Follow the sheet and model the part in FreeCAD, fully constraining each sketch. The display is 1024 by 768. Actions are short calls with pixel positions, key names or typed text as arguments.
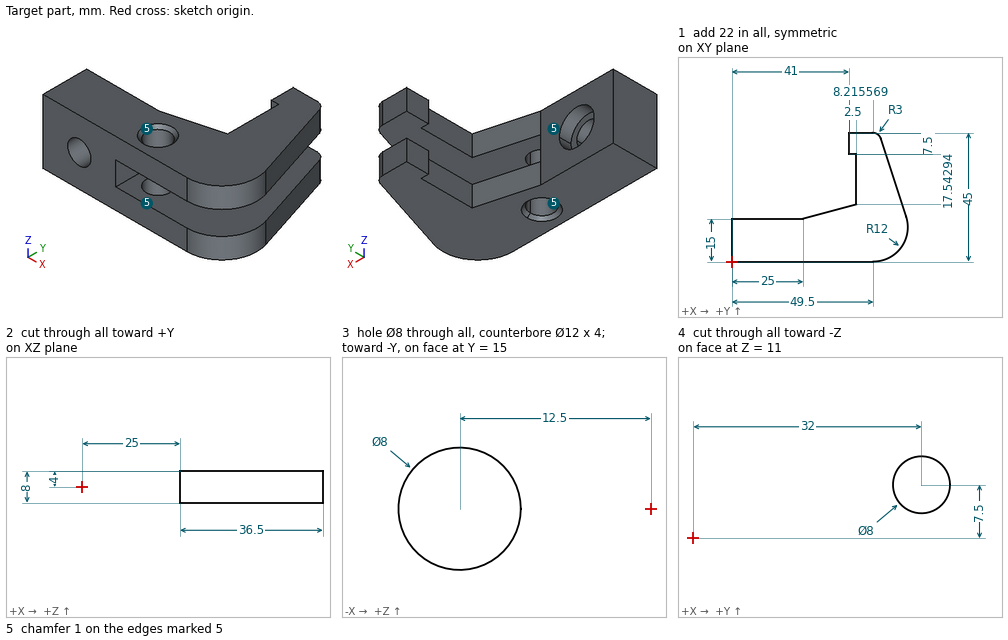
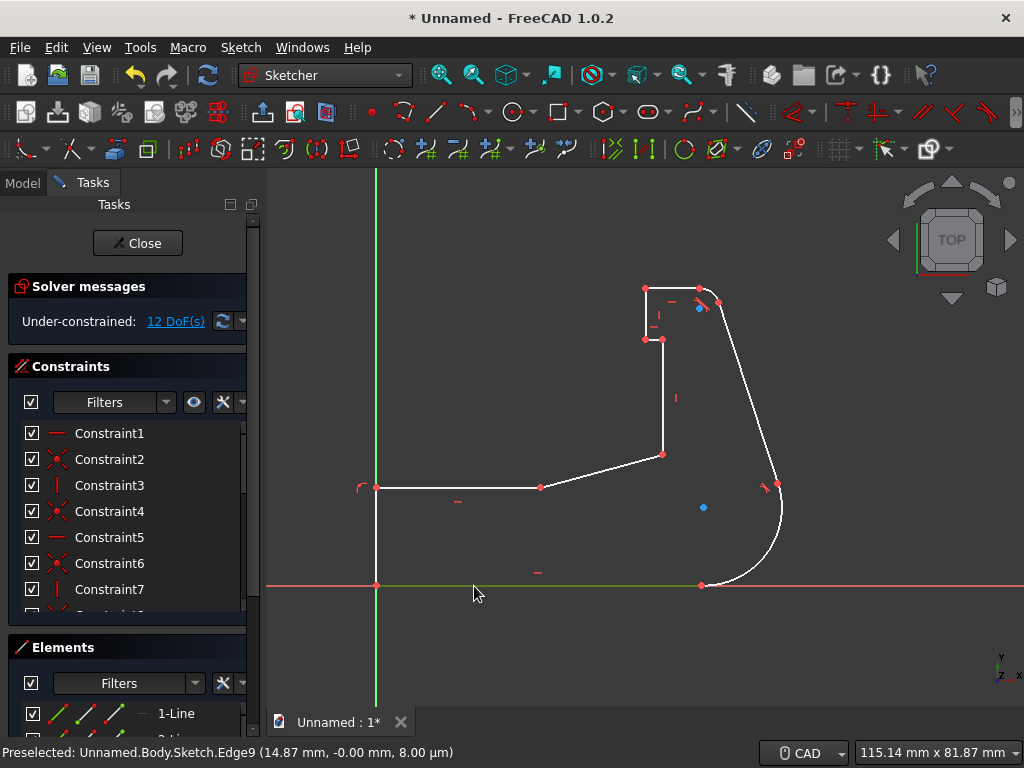
click(745, 574)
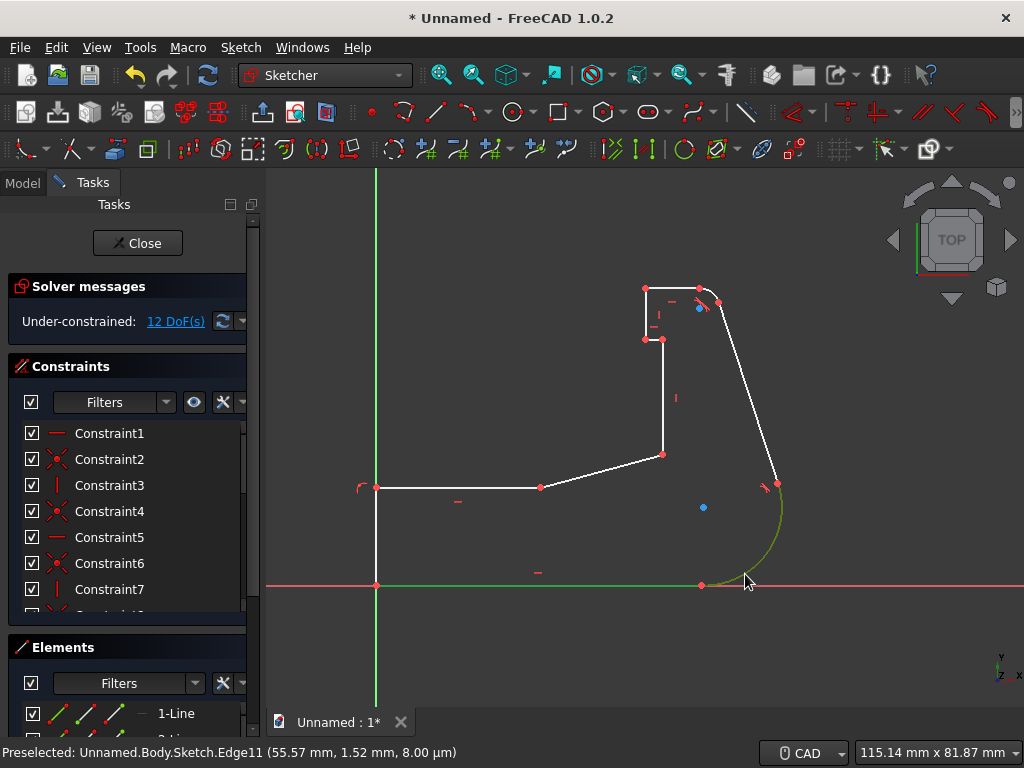
key(t)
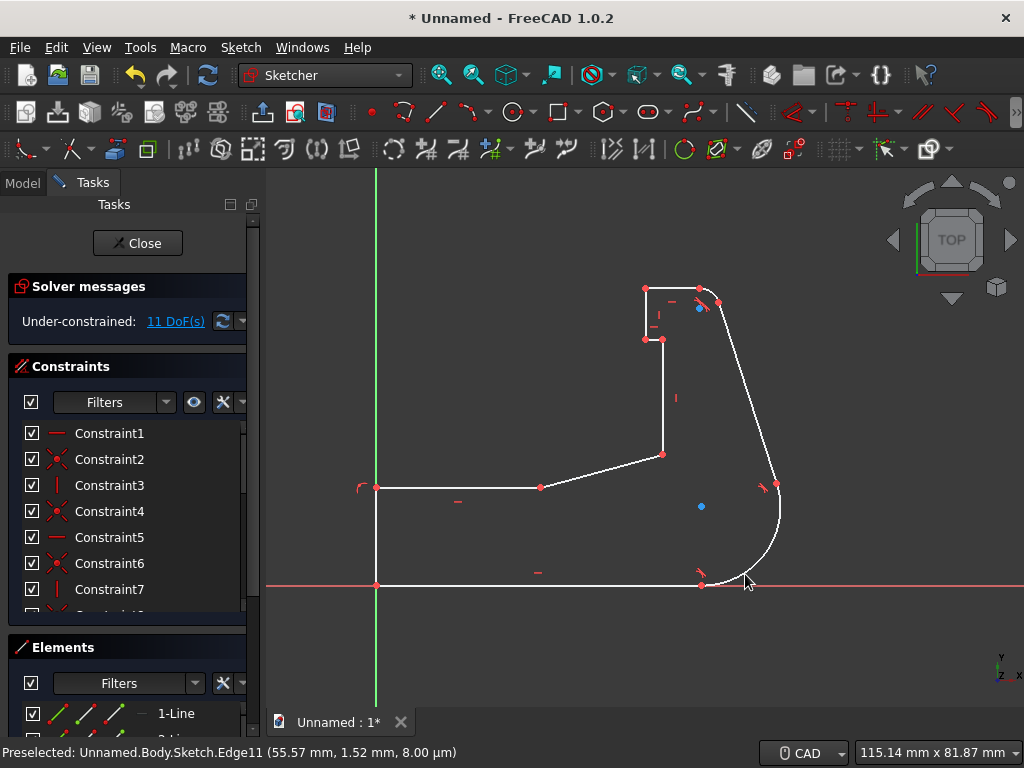
click(792, 112)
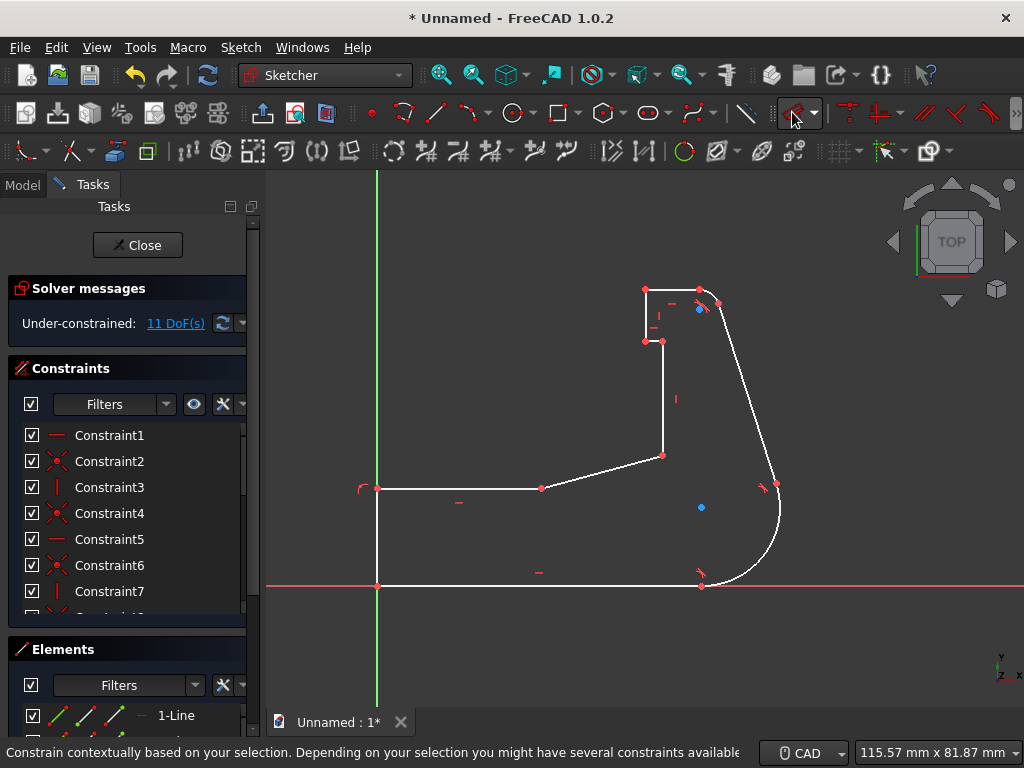
scroll(711, 294, up, 4)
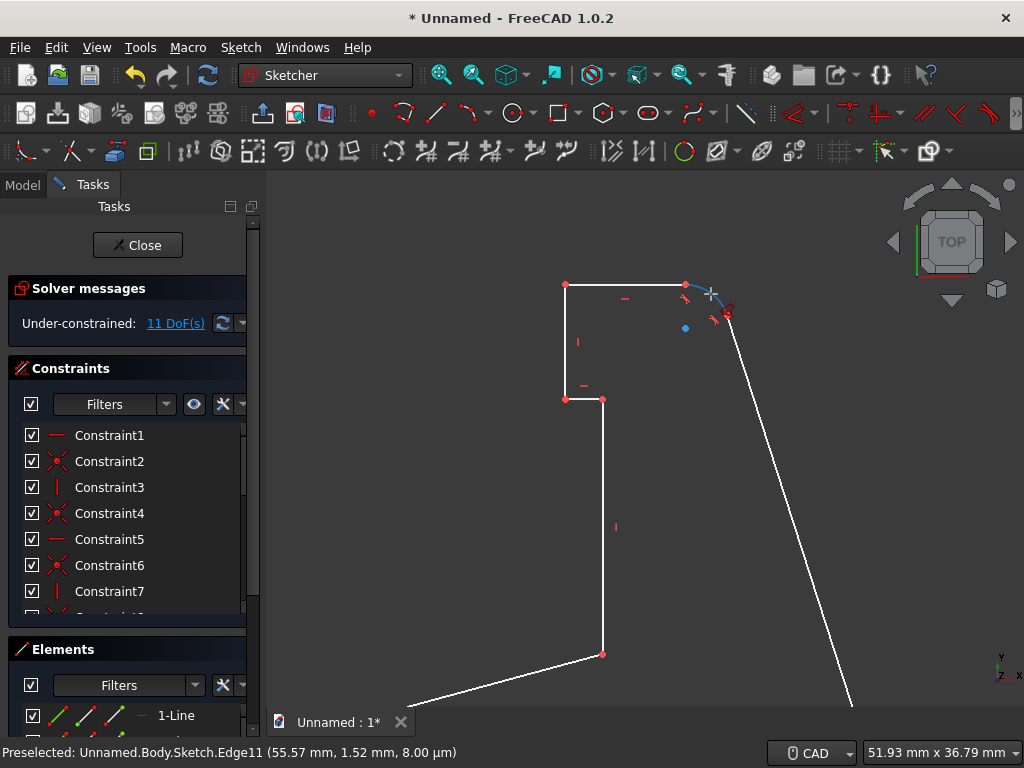
click(711, 293)
click(730, 267)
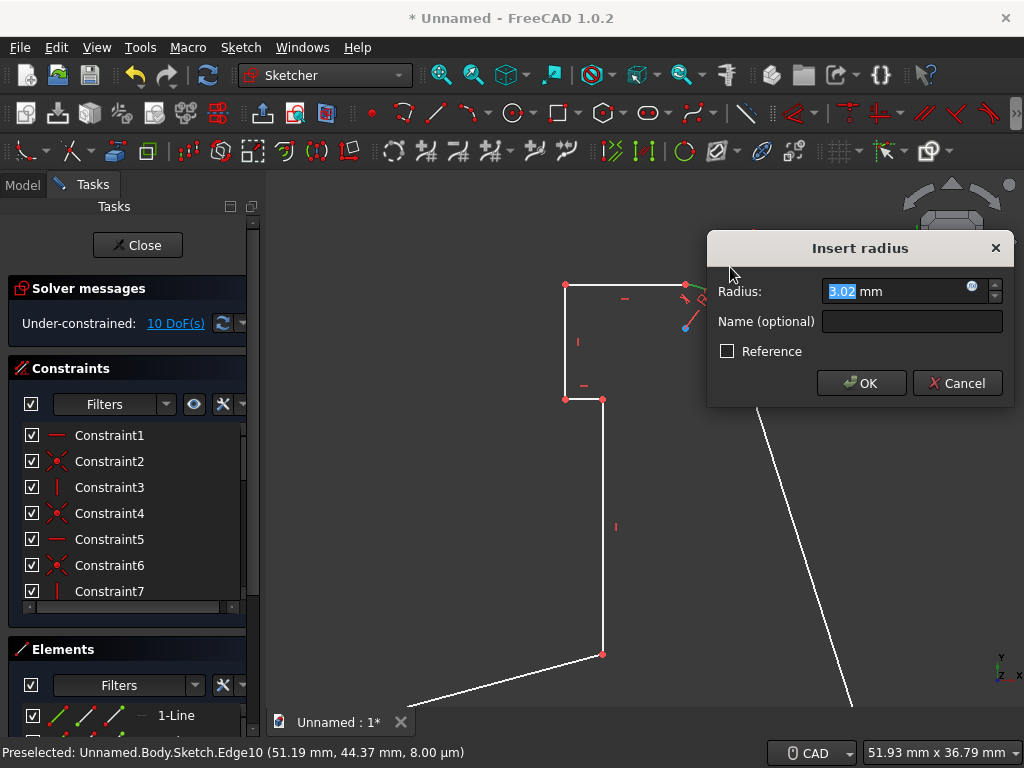
text(3)
key(Return)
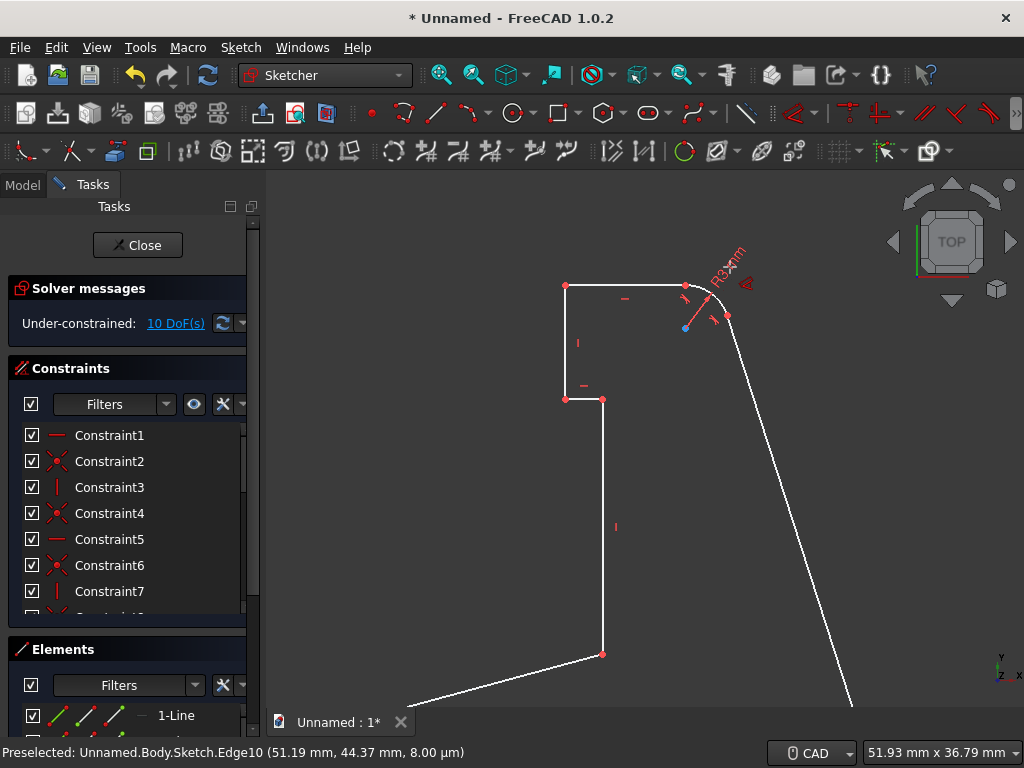
scroll(711, 294, down, 4)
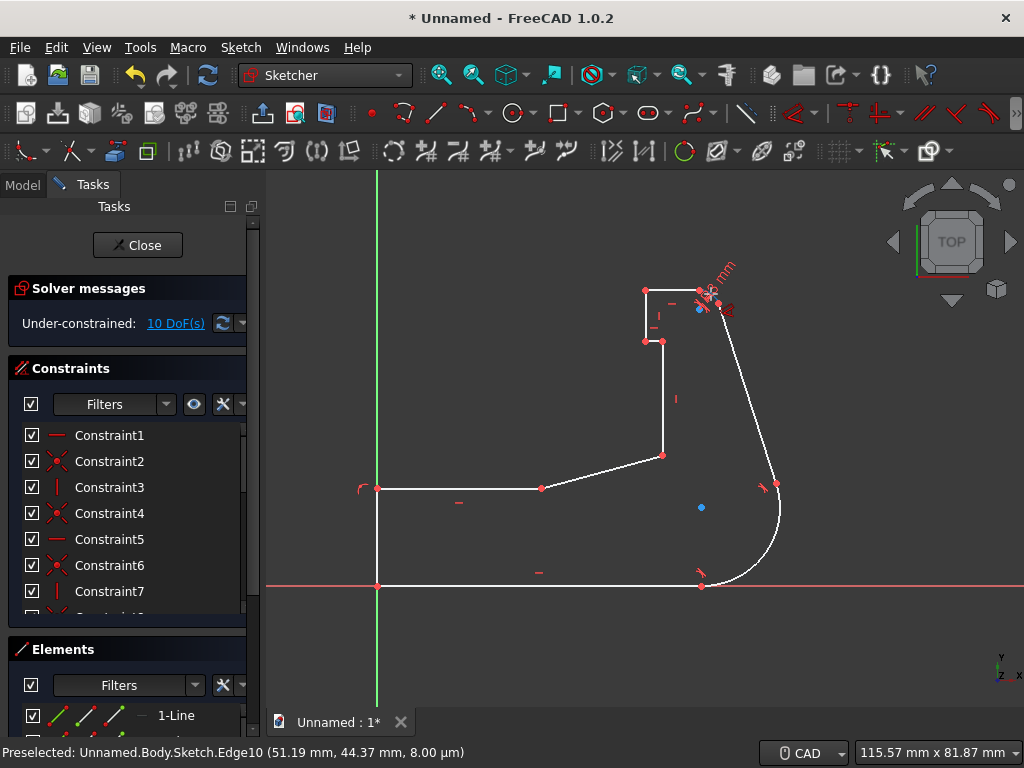
click(743, 574)
click(760, 601)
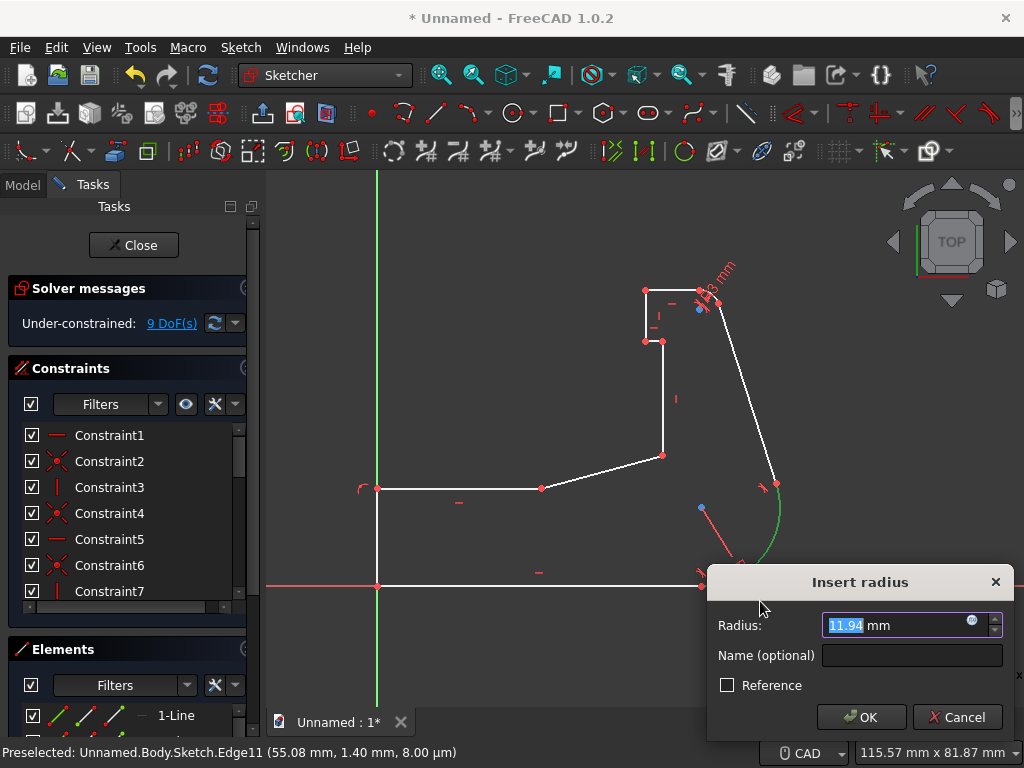
text(12)
key(Return)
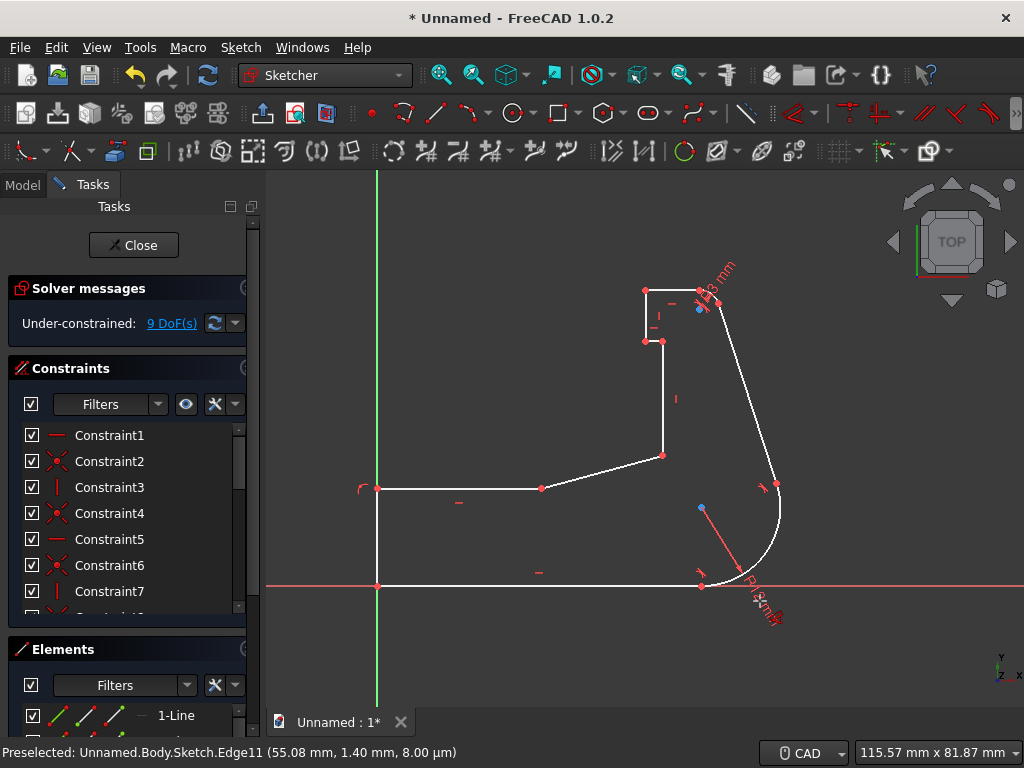
click(492, 489)
click(459, 523)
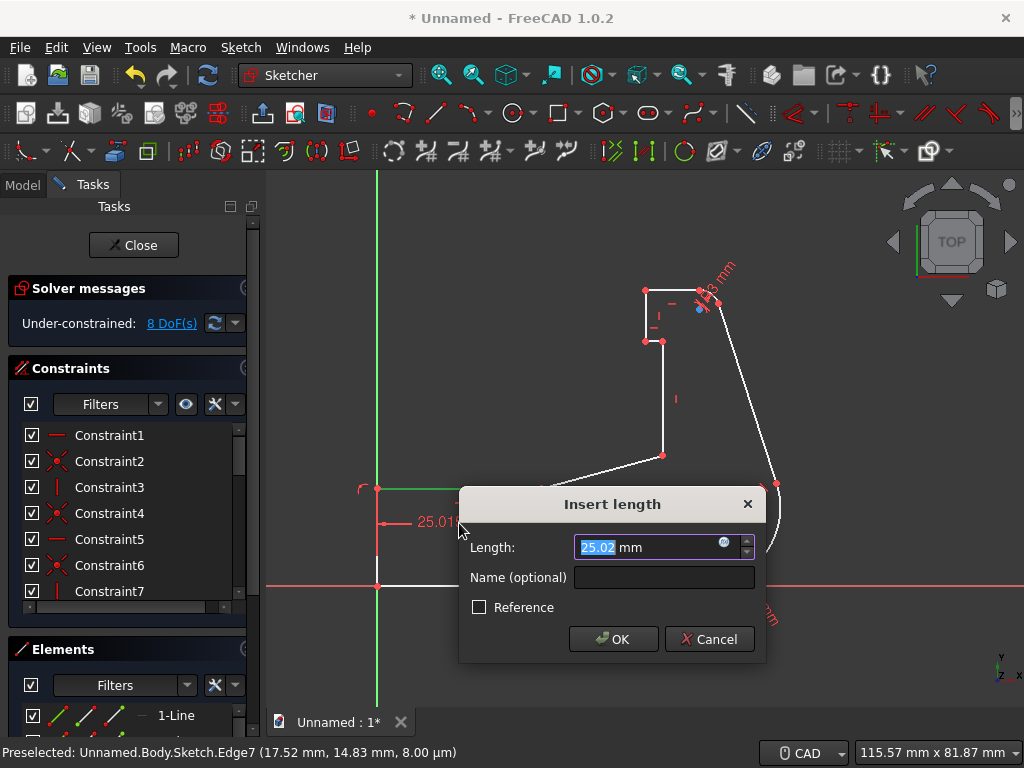
text(25)
key(Return)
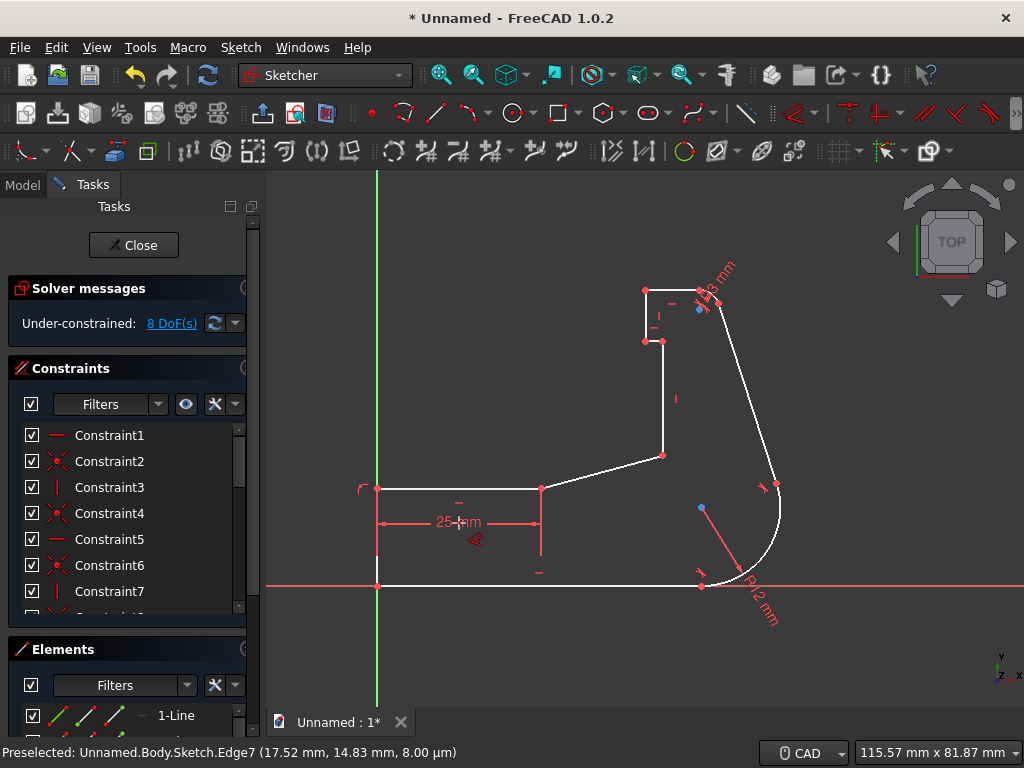
click(377, 518)
click(343, 537)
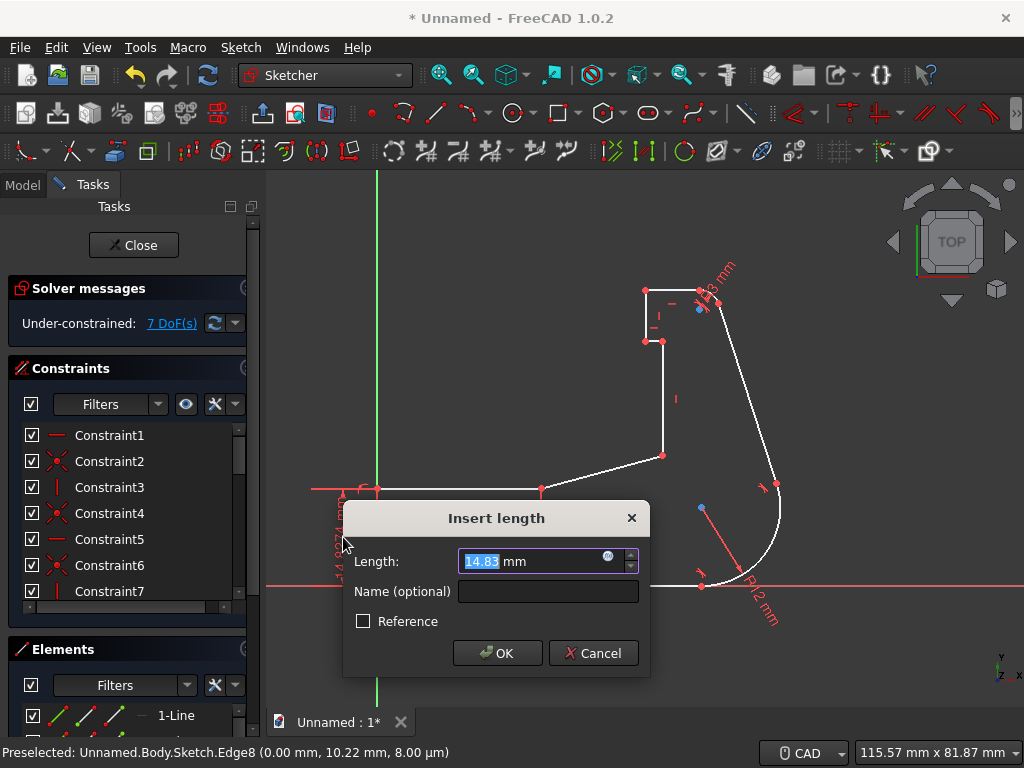
text(15)
key(Return)